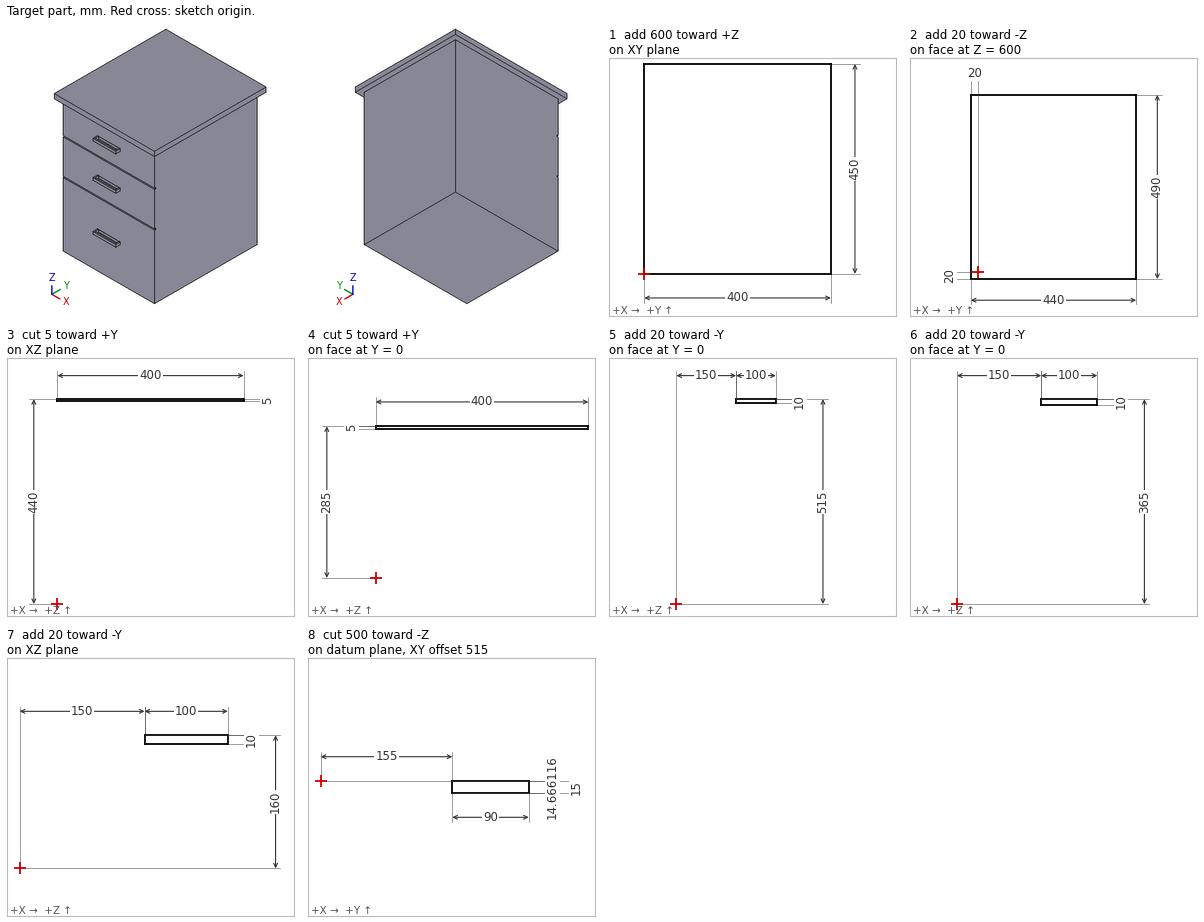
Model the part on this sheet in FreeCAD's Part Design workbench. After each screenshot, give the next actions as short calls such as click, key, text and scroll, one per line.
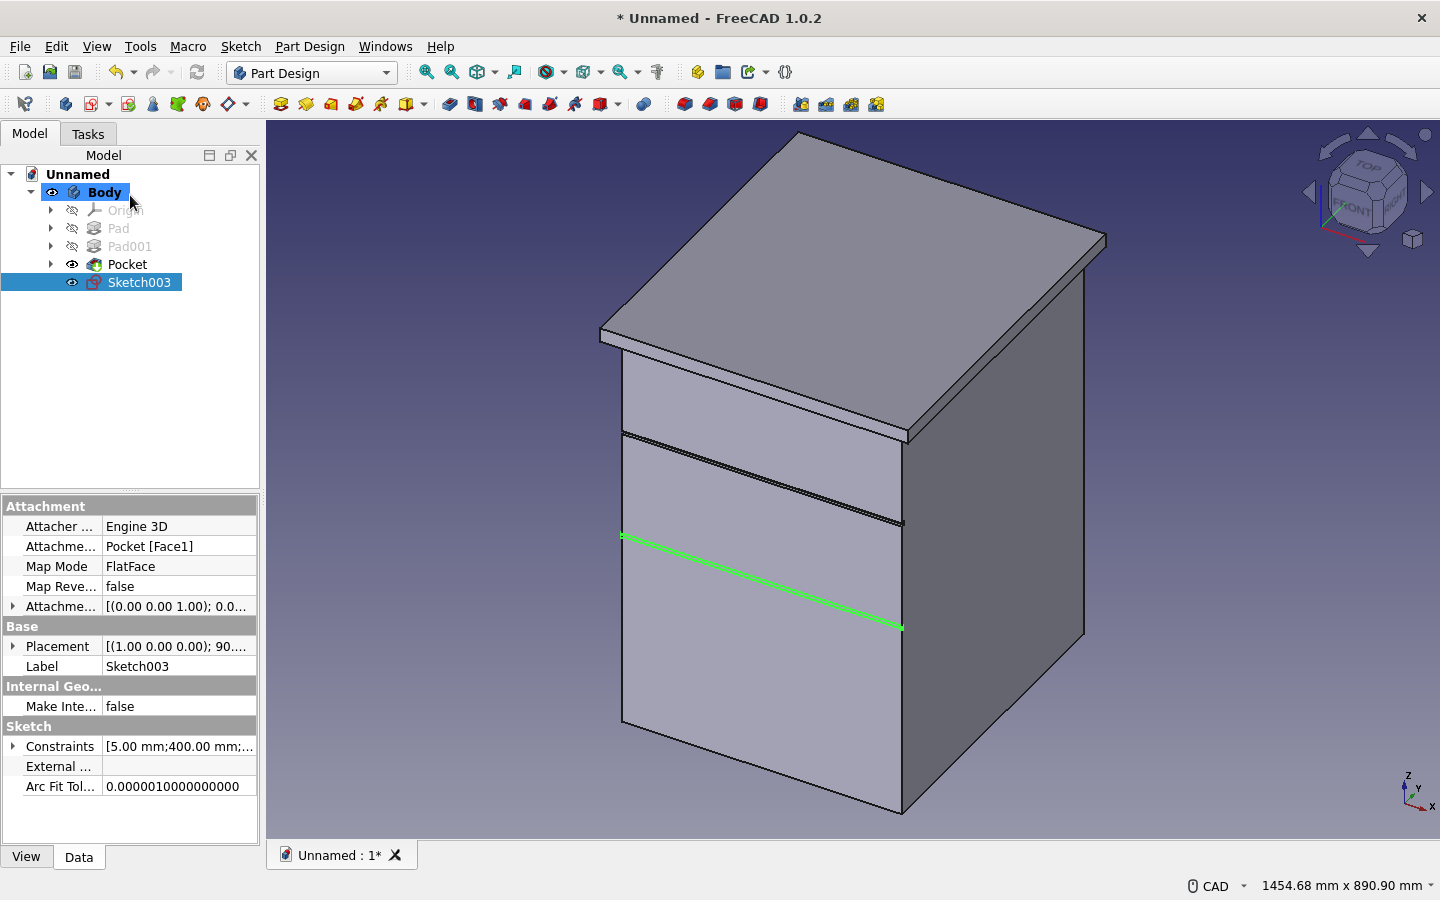
click(450, 104)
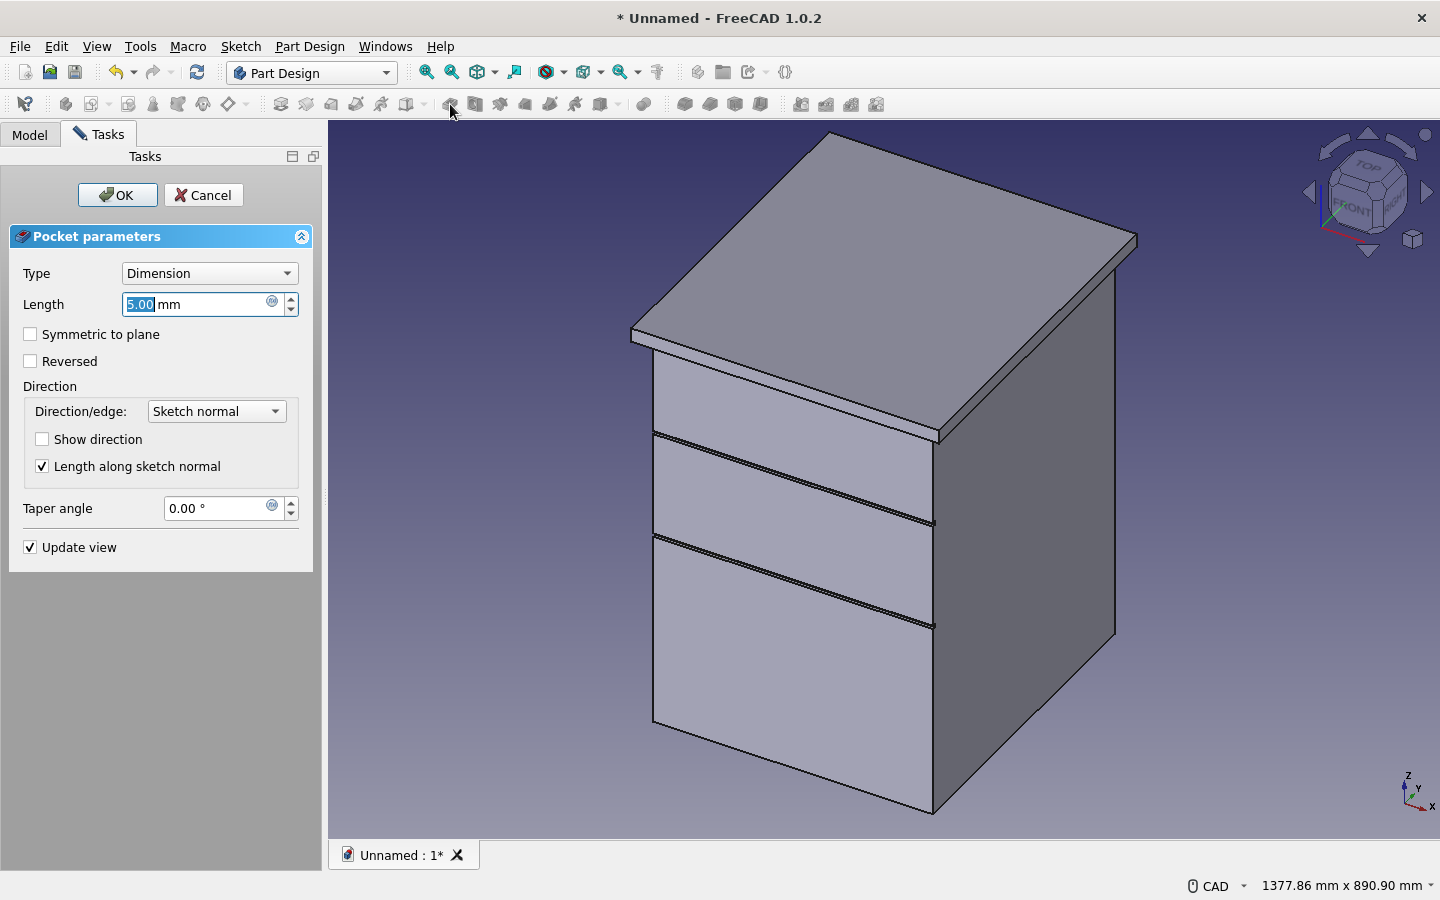
text(5)
key(Tab)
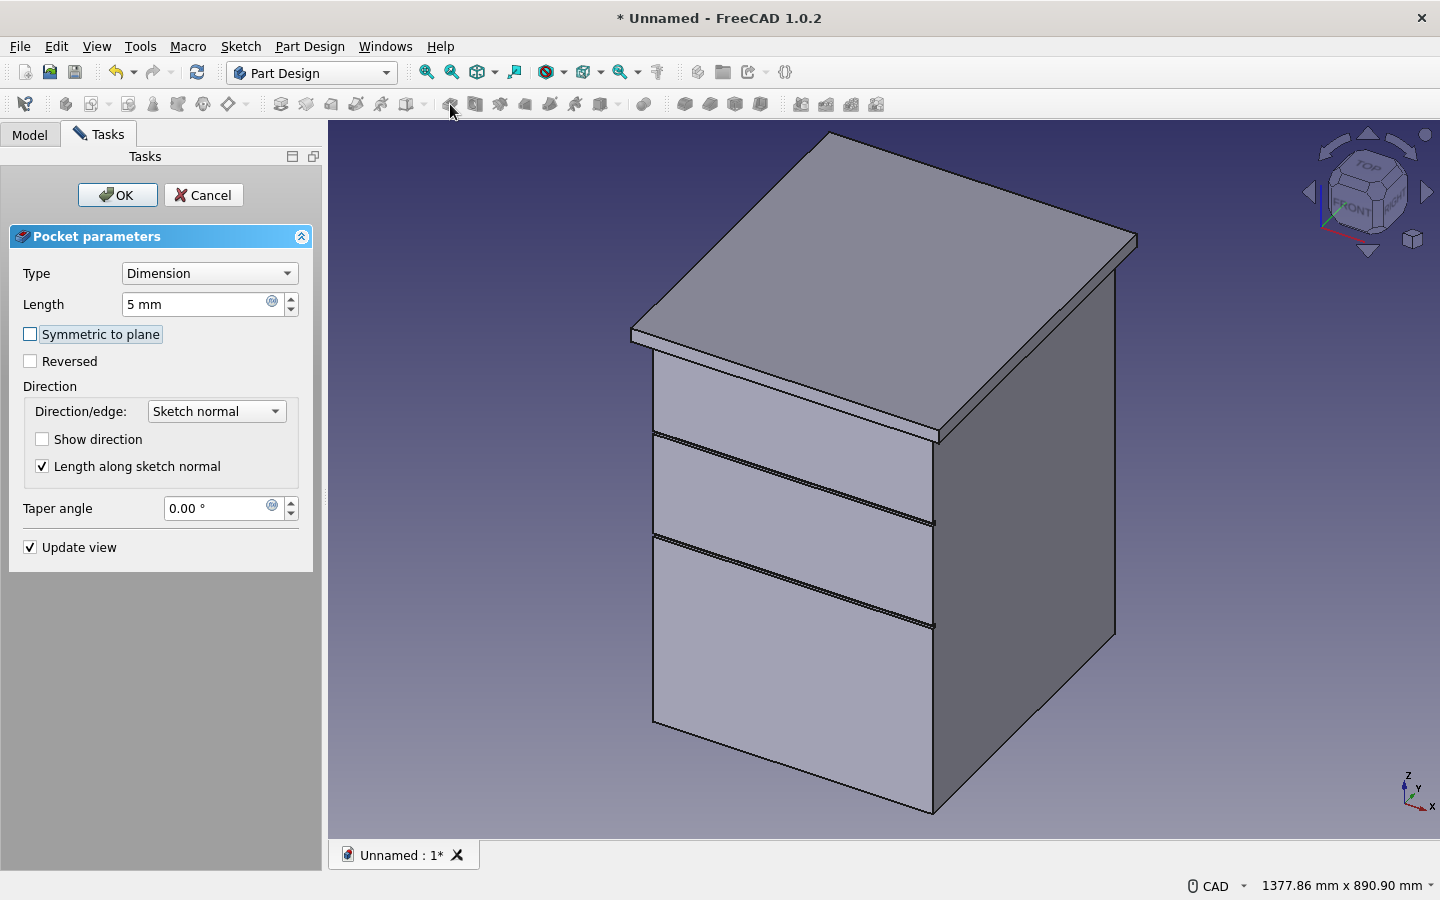
click(118, 195)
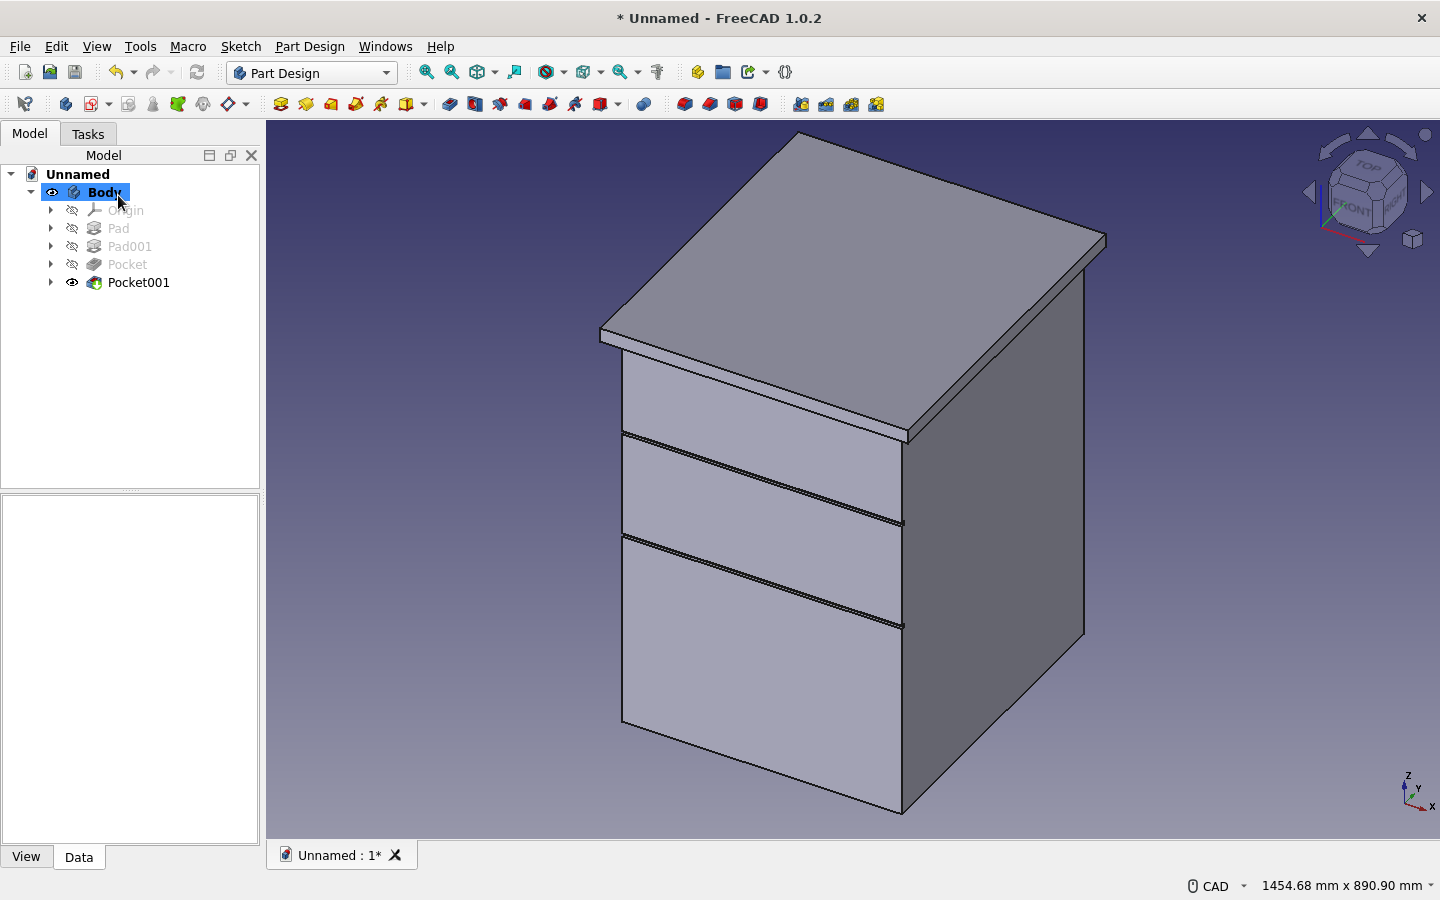
click(802, 688)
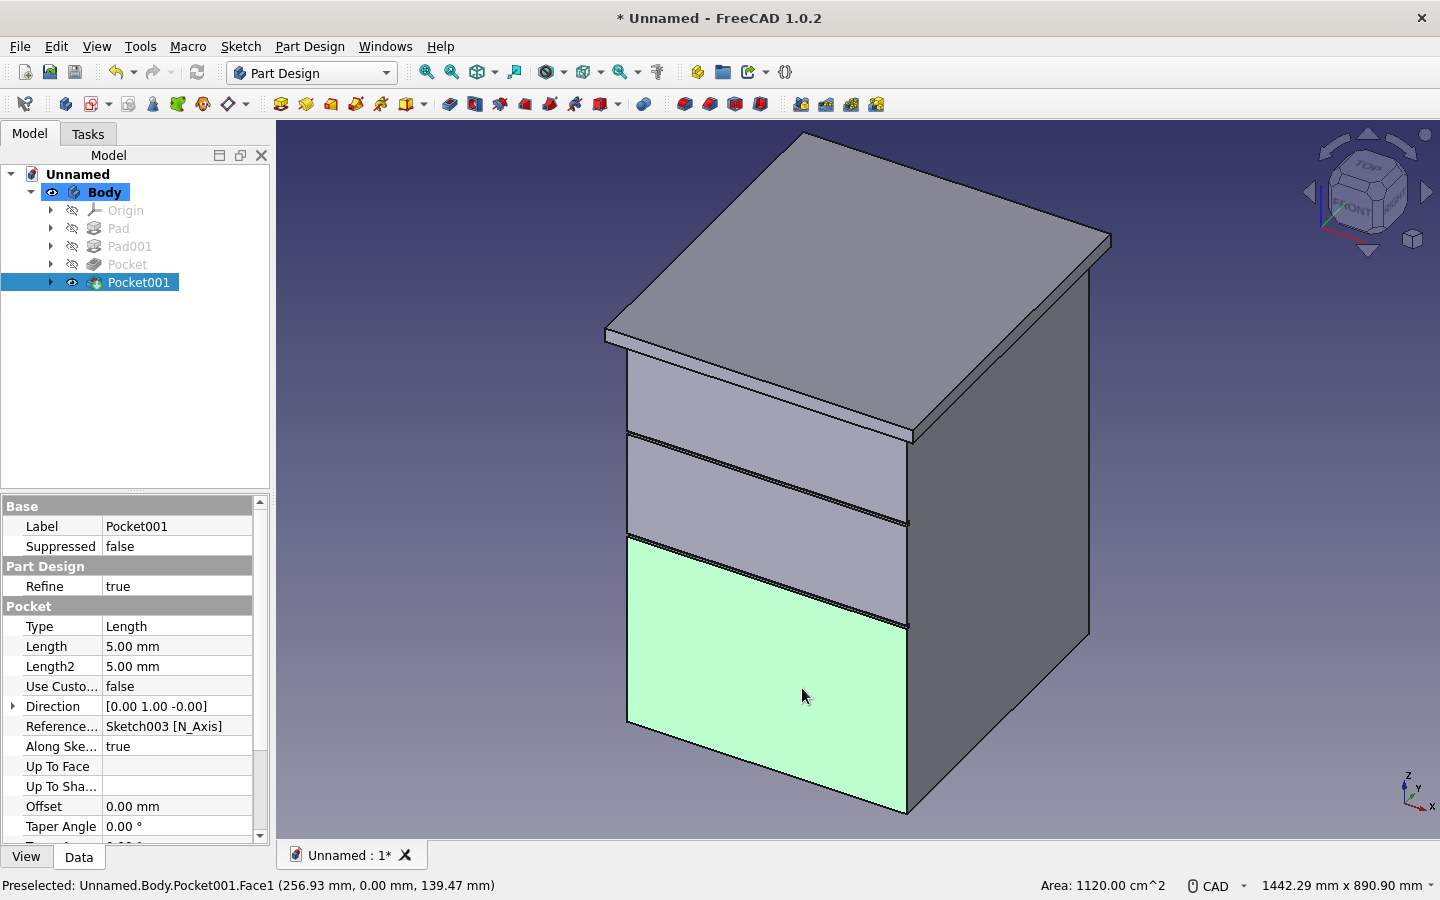
click(90, 104)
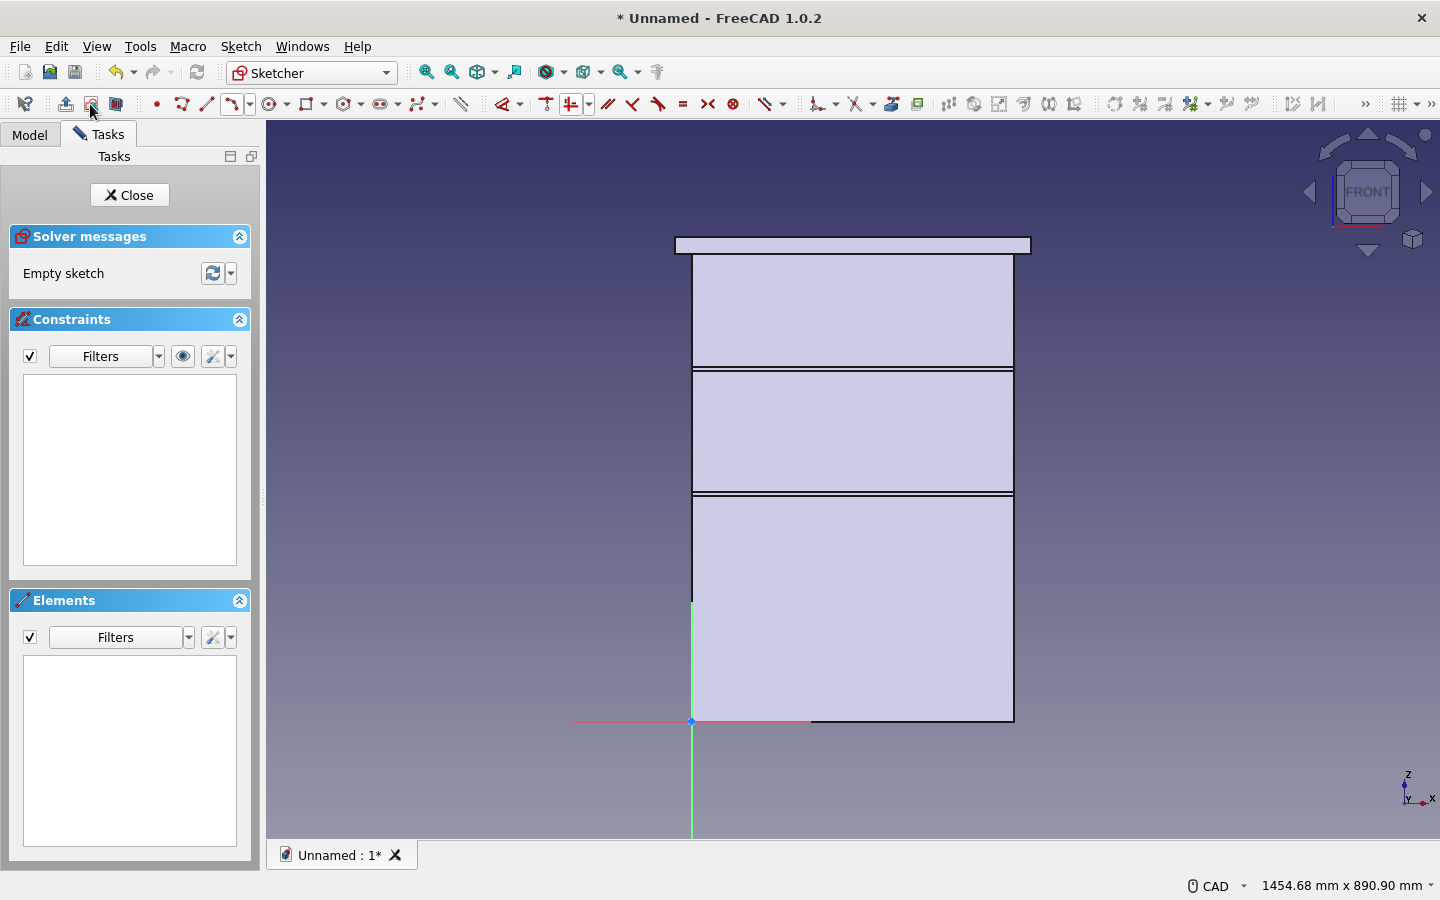
click(116, 104)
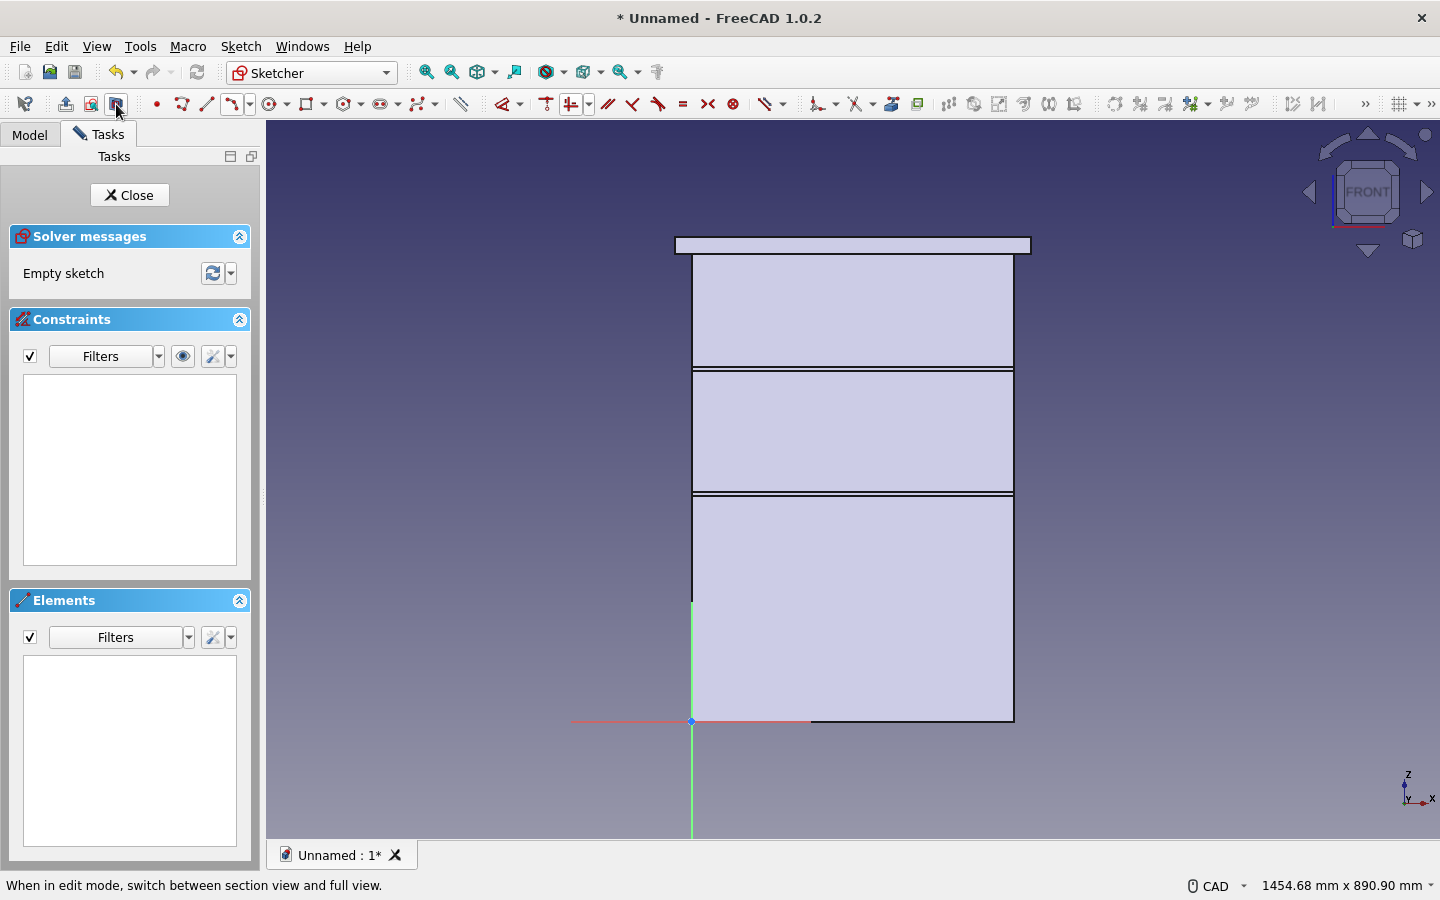
scroll(862, 289, up, 11)